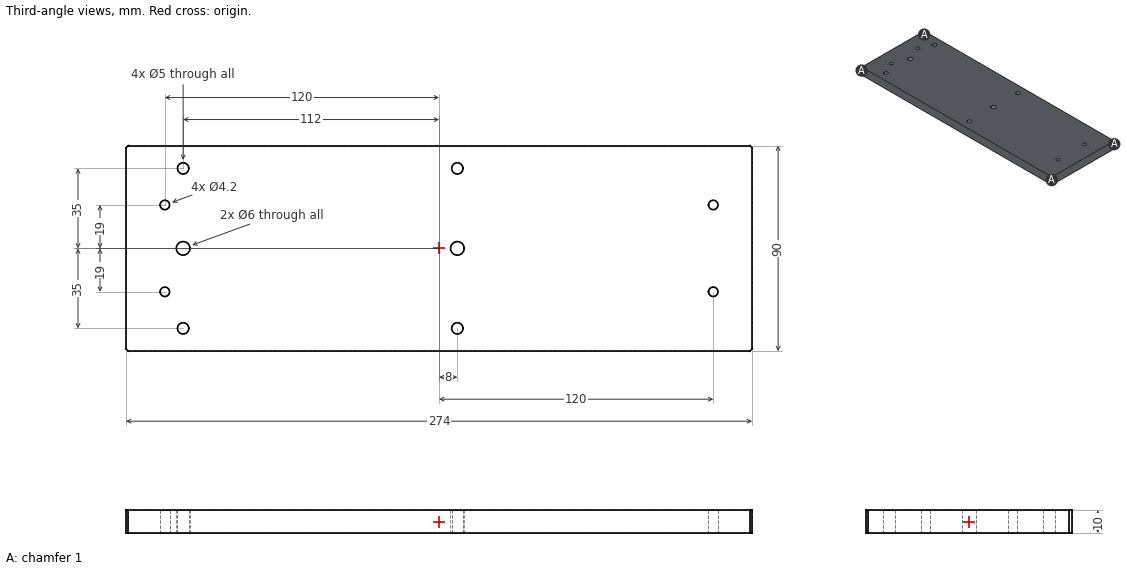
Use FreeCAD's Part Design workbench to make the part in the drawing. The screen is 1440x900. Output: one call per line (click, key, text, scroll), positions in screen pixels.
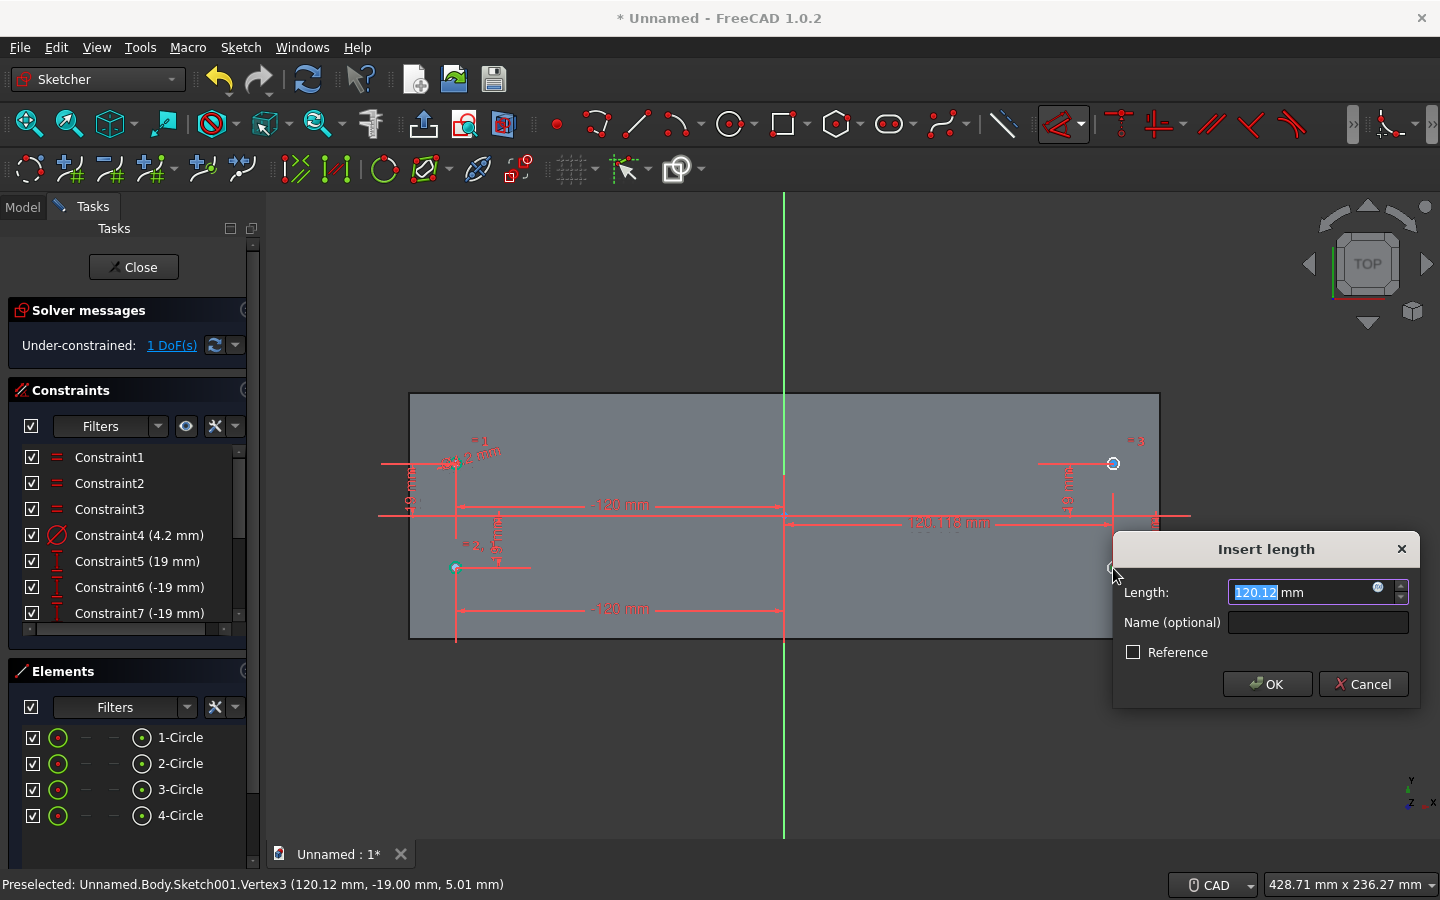
text(120)
key(Return)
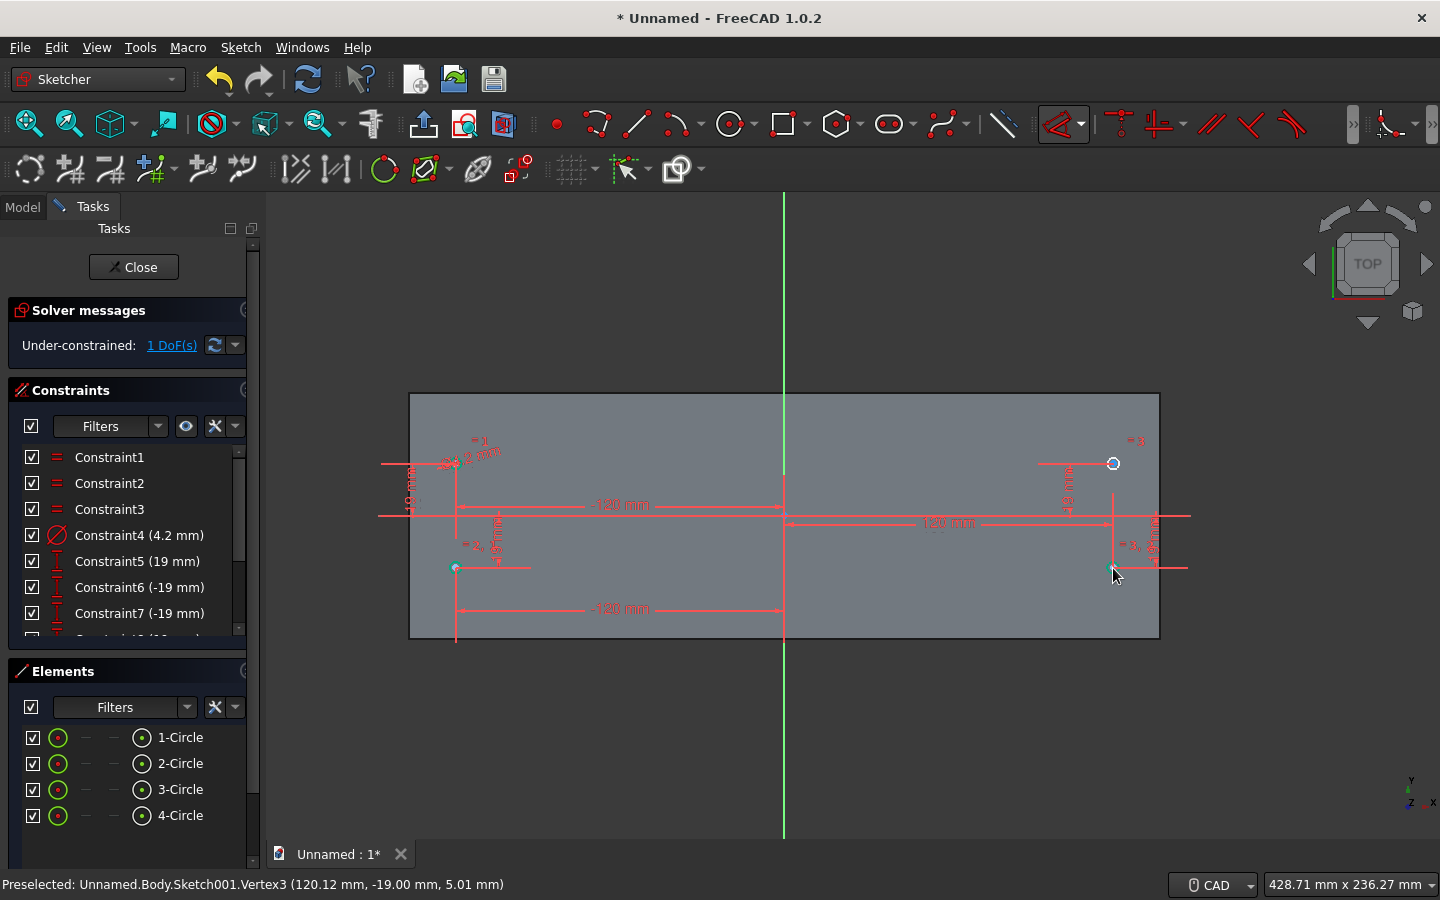
click(1113, 464)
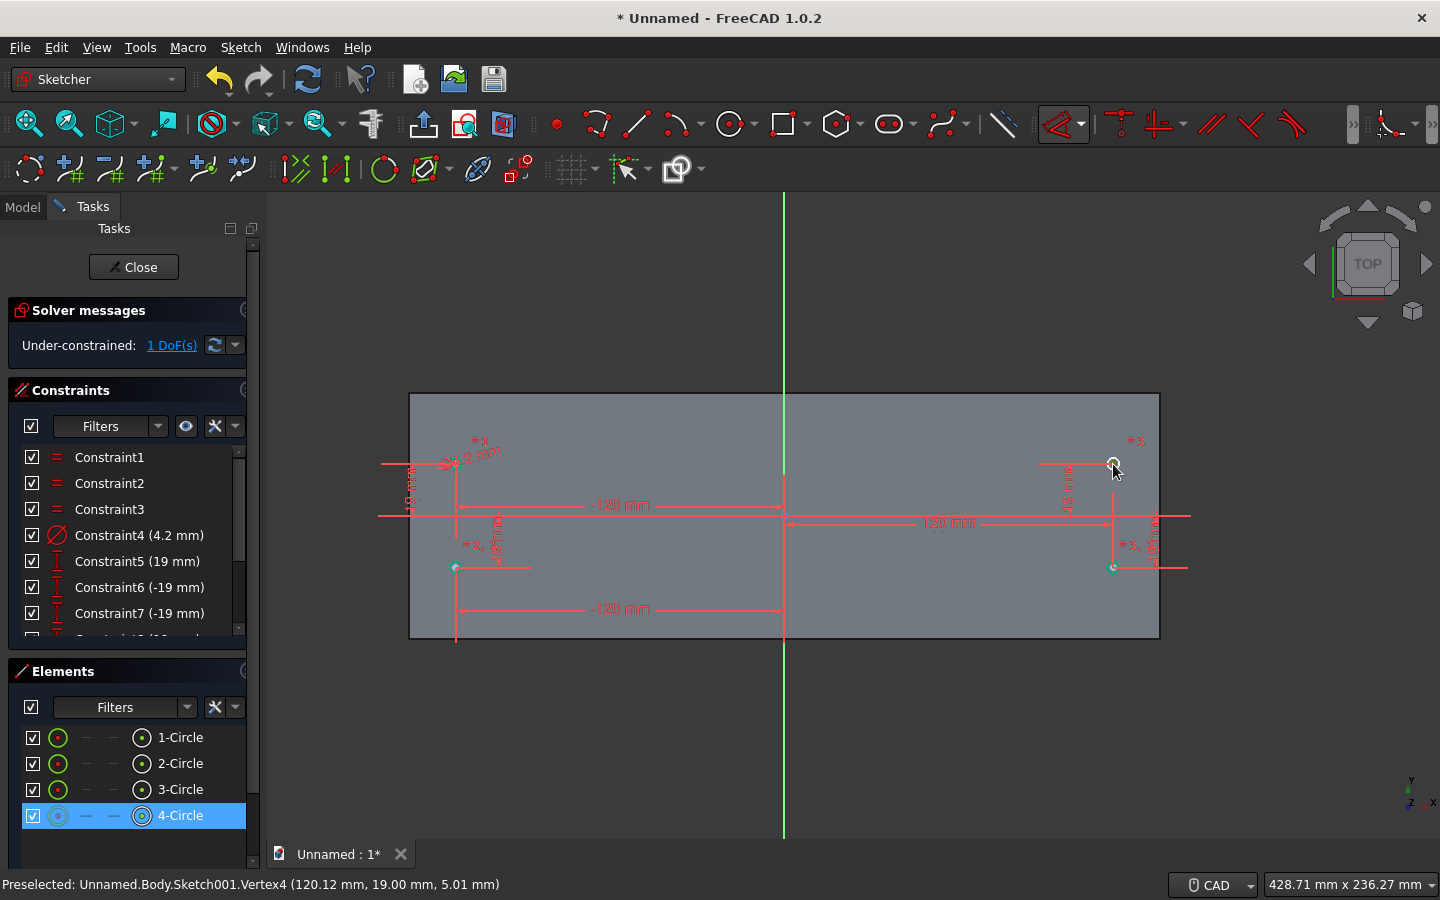
key(l)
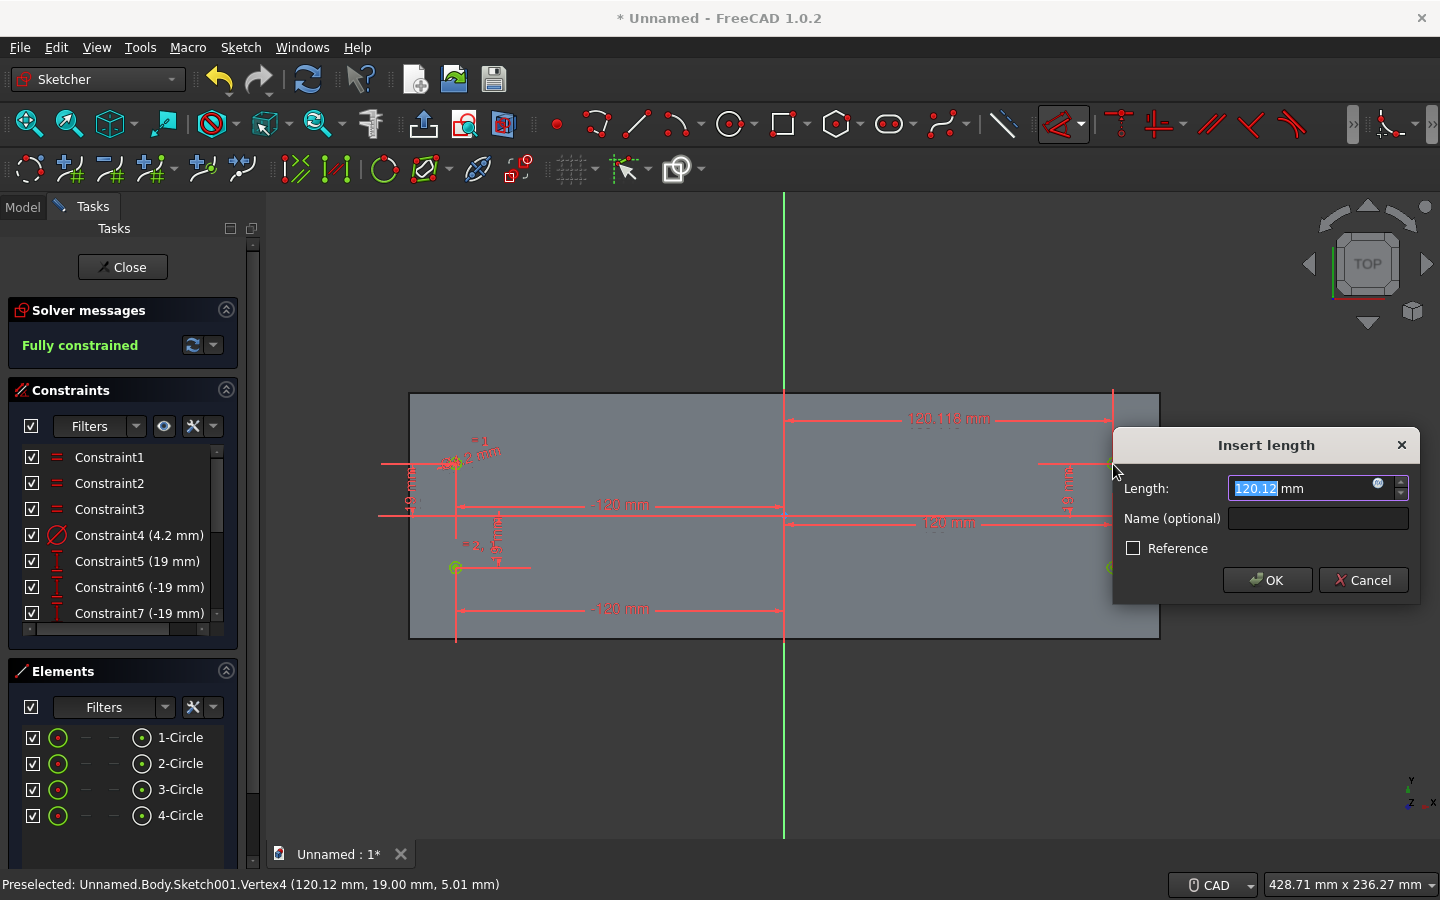
text(120)
key(Return)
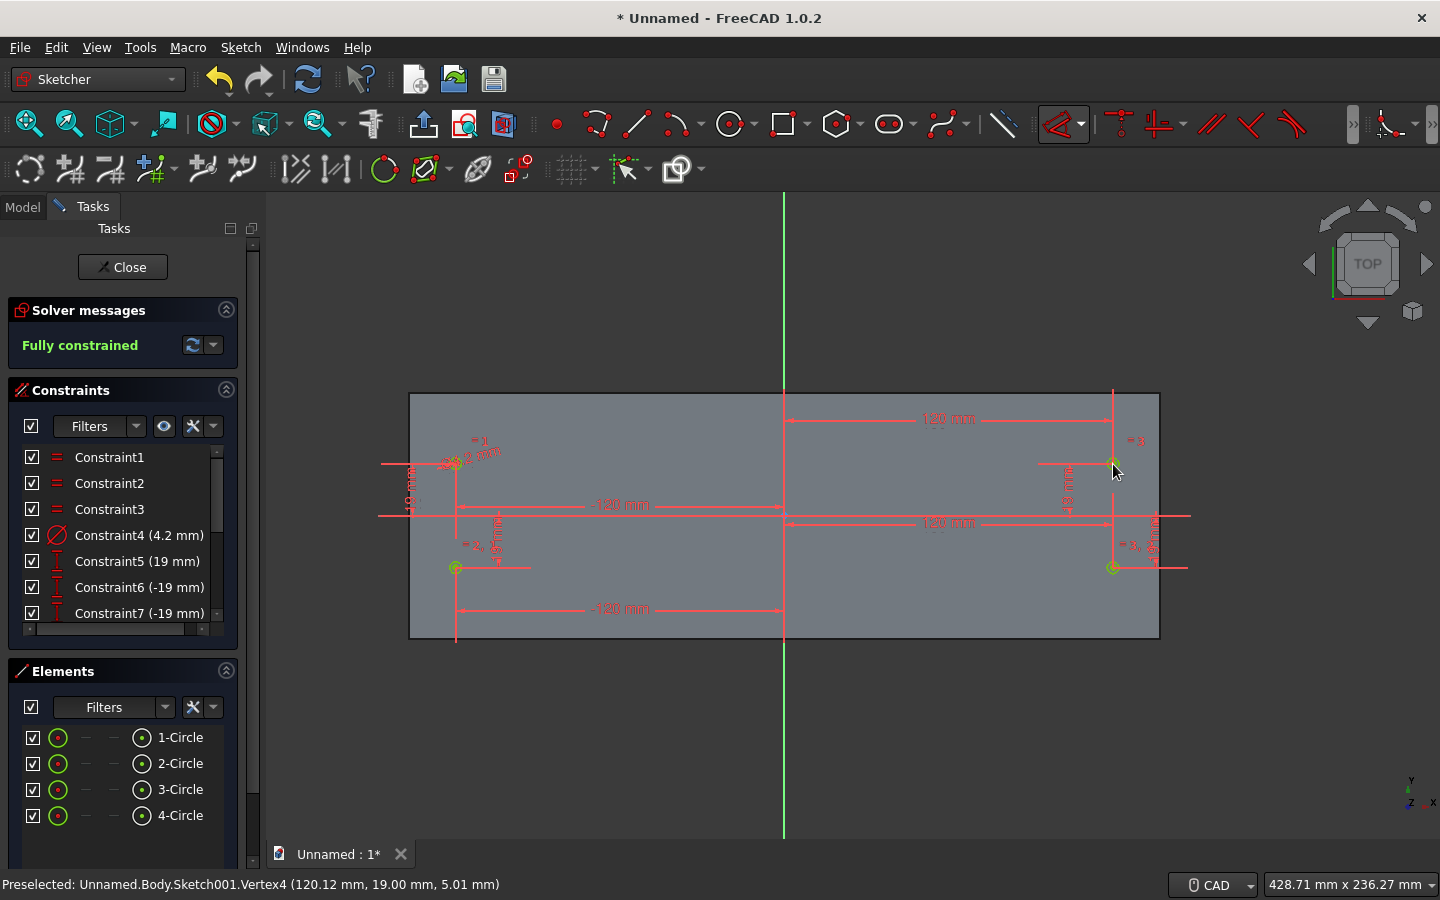
click(123, 267)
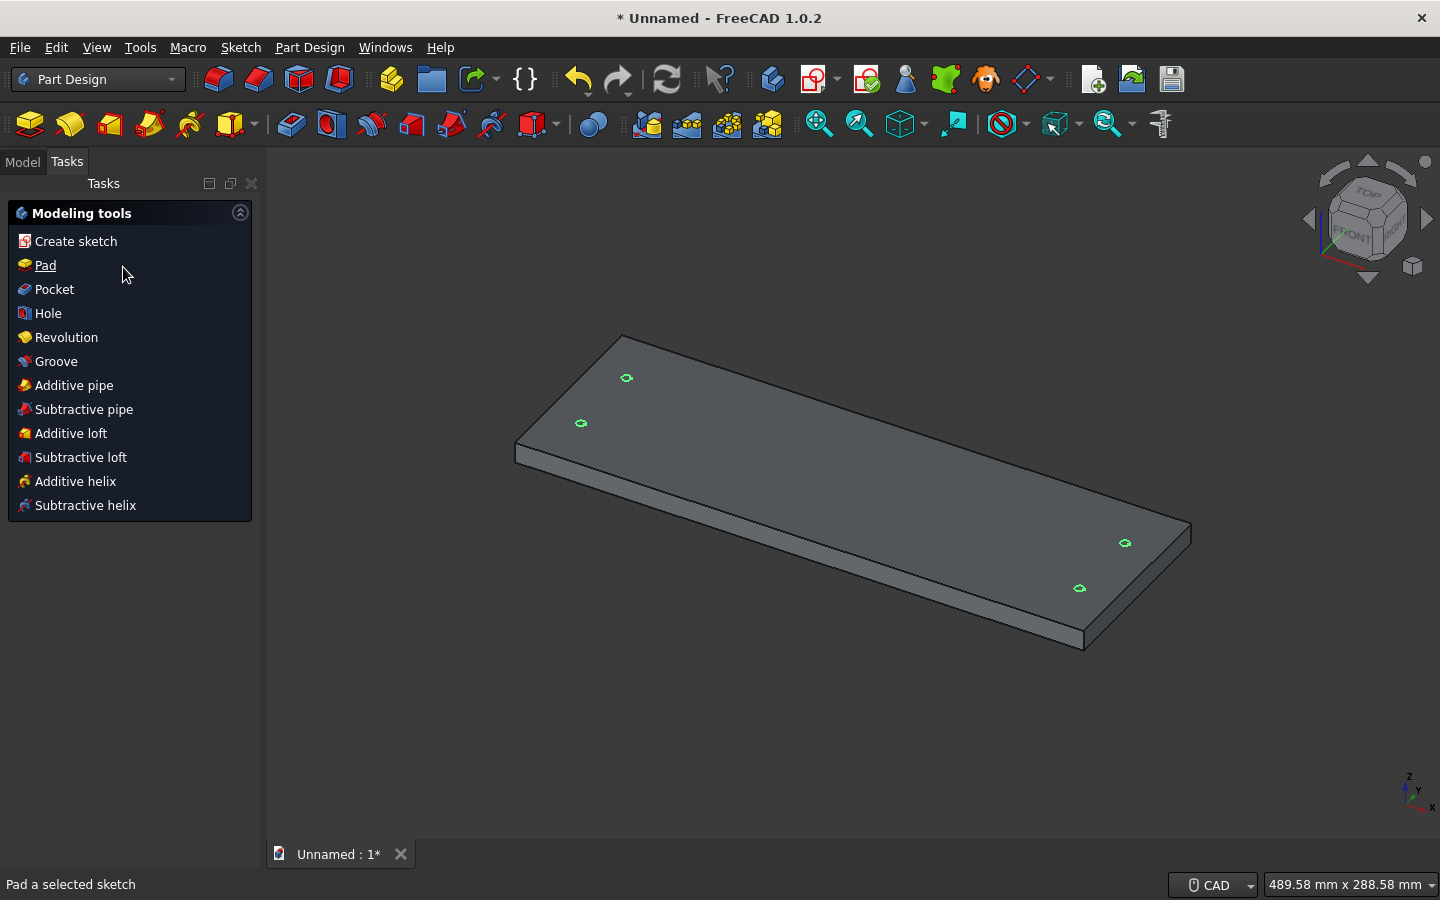
click(292, 124)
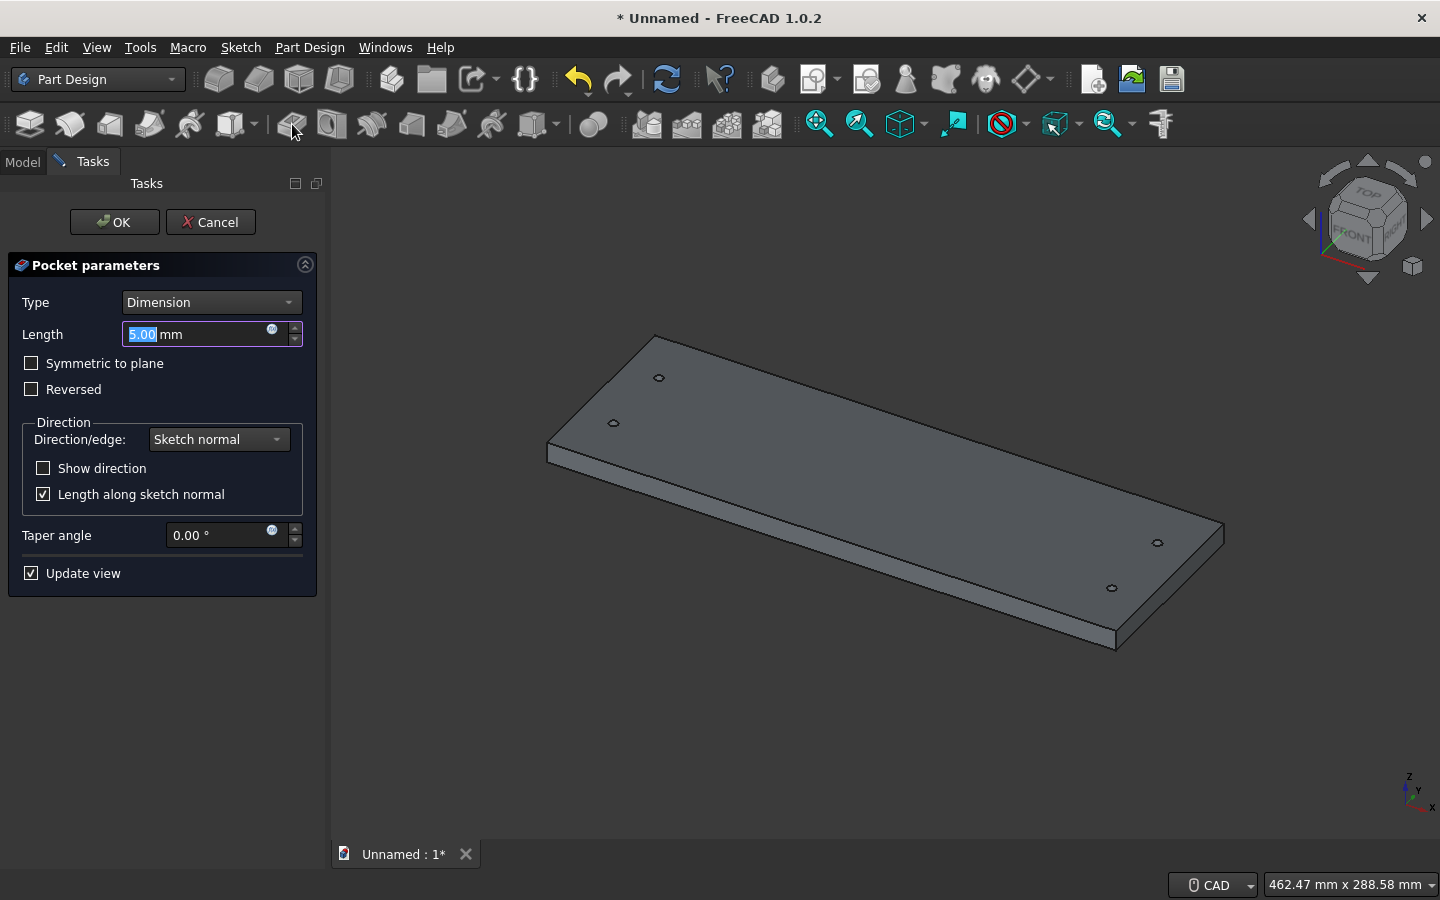
click(212, 302)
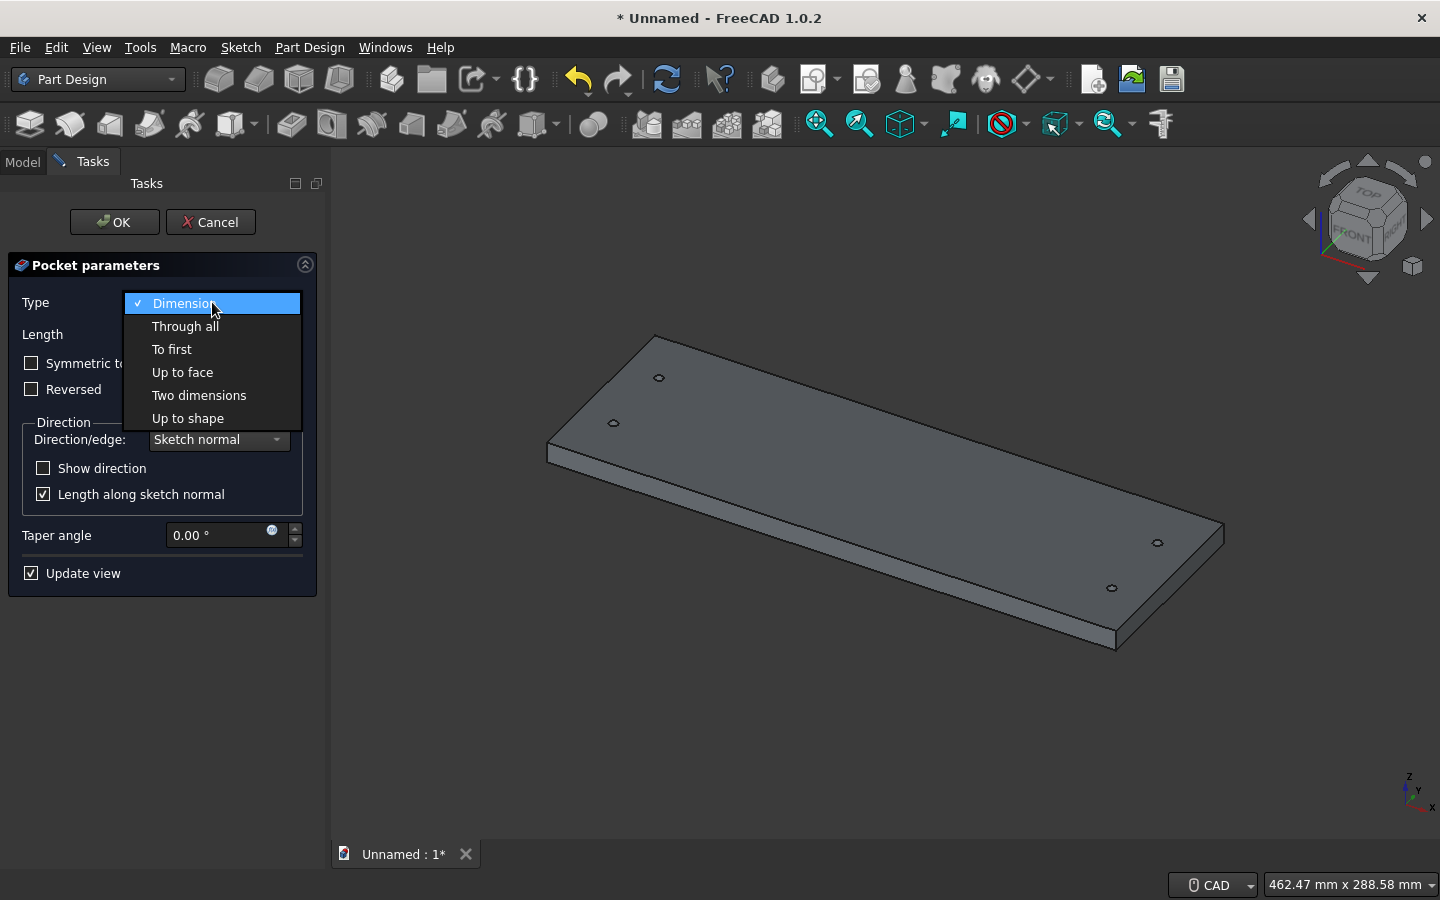
click(212, 326)